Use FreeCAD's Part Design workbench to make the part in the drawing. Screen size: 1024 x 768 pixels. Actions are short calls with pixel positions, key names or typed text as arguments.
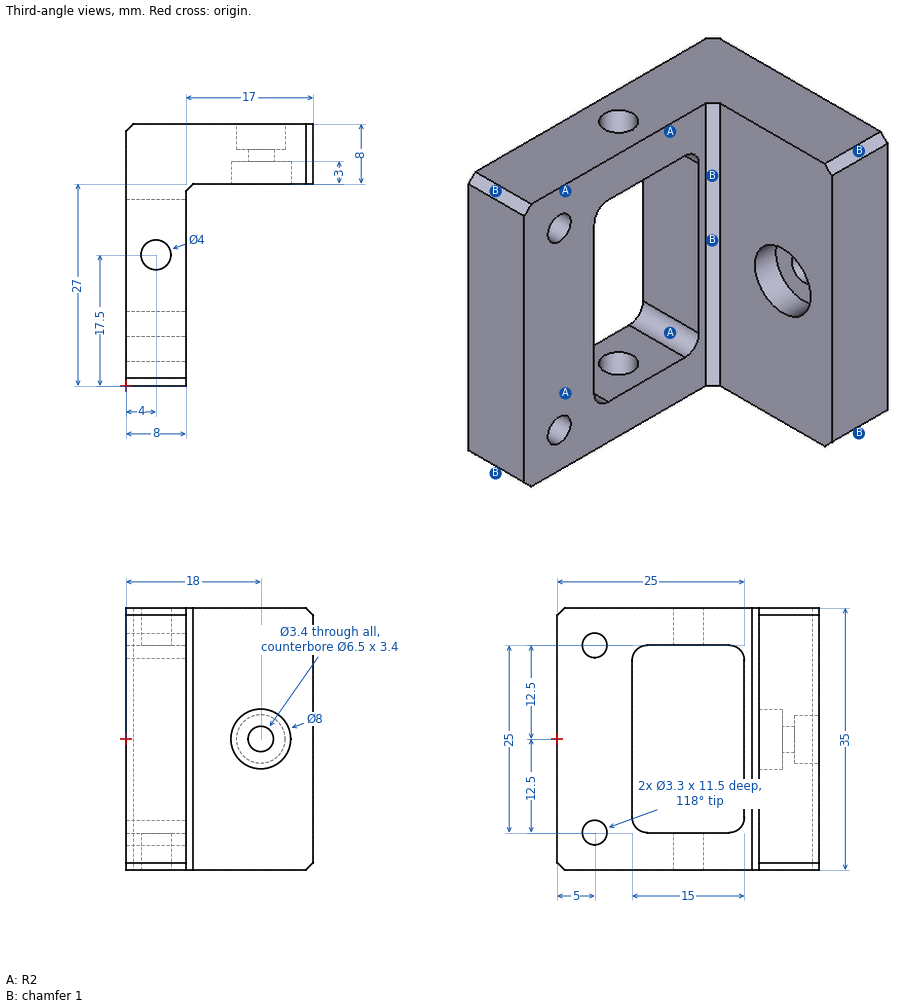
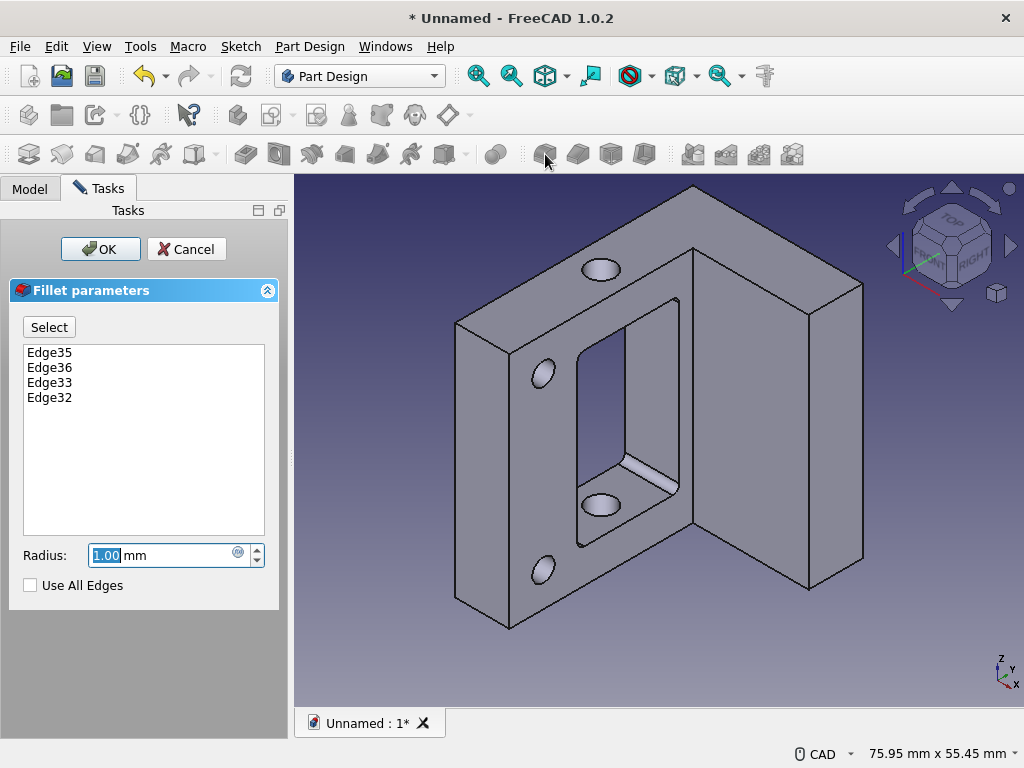
text(2)
key(Tab)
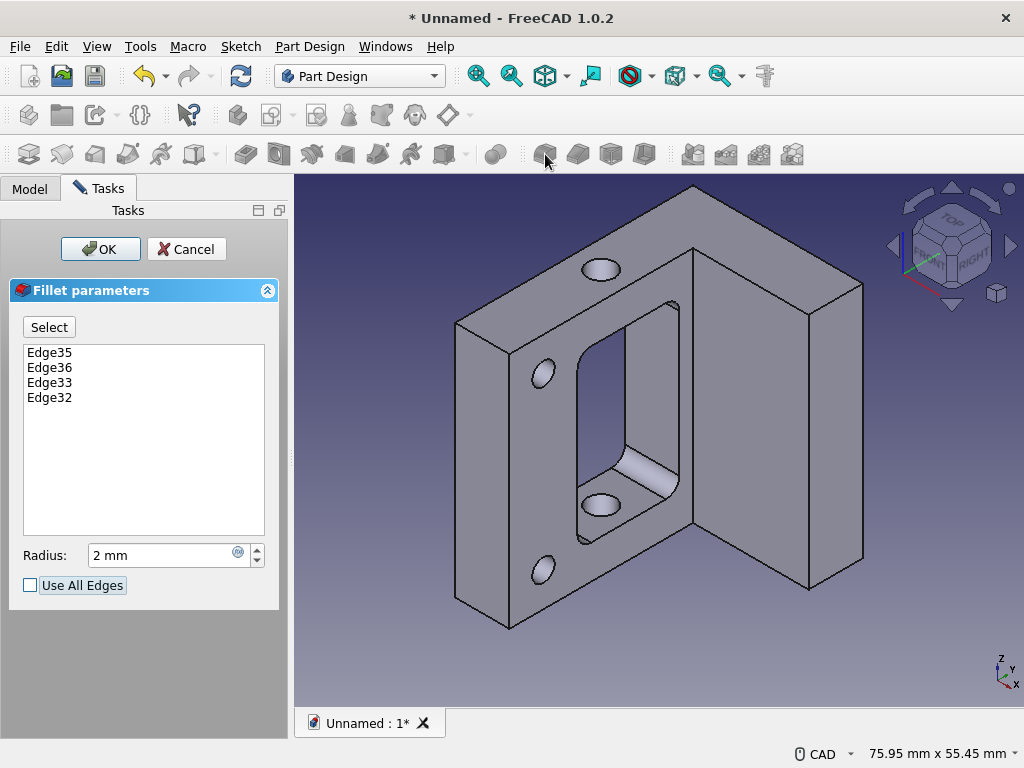
click(101, 249)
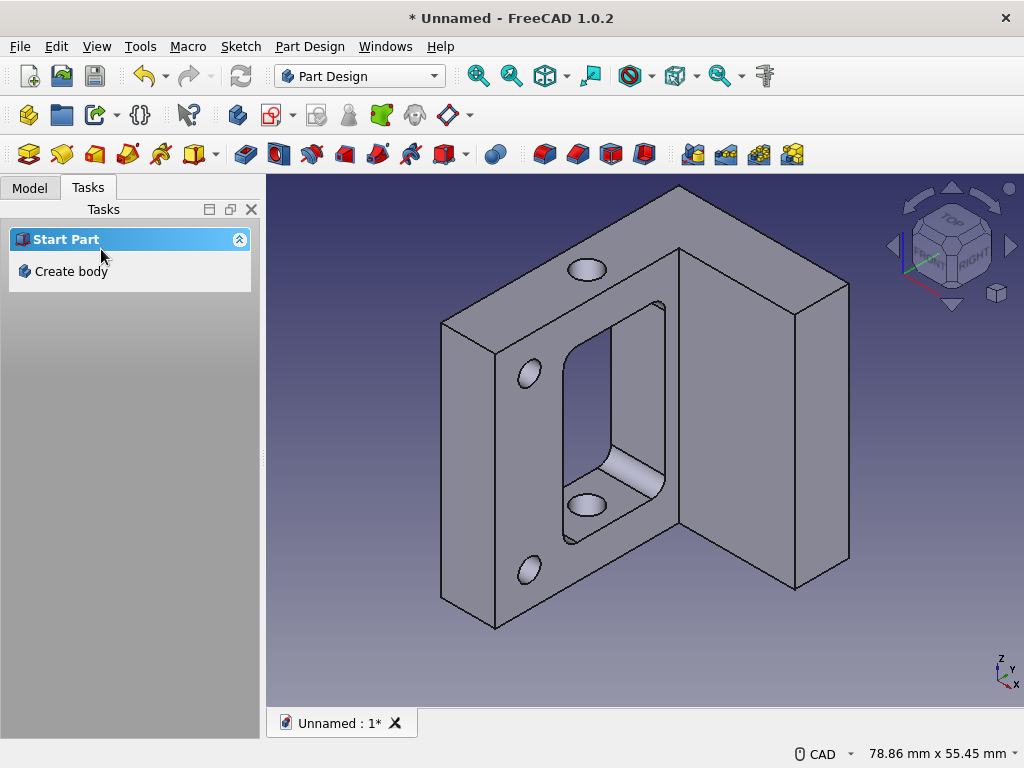
click(737, 379)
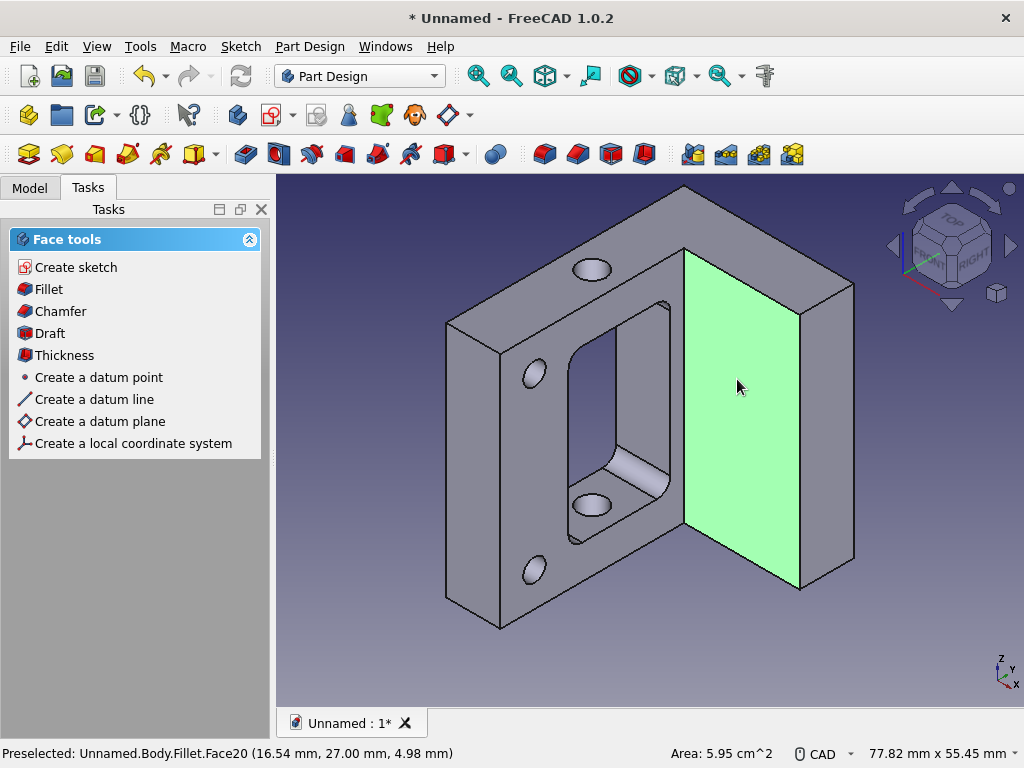
click(270, 116)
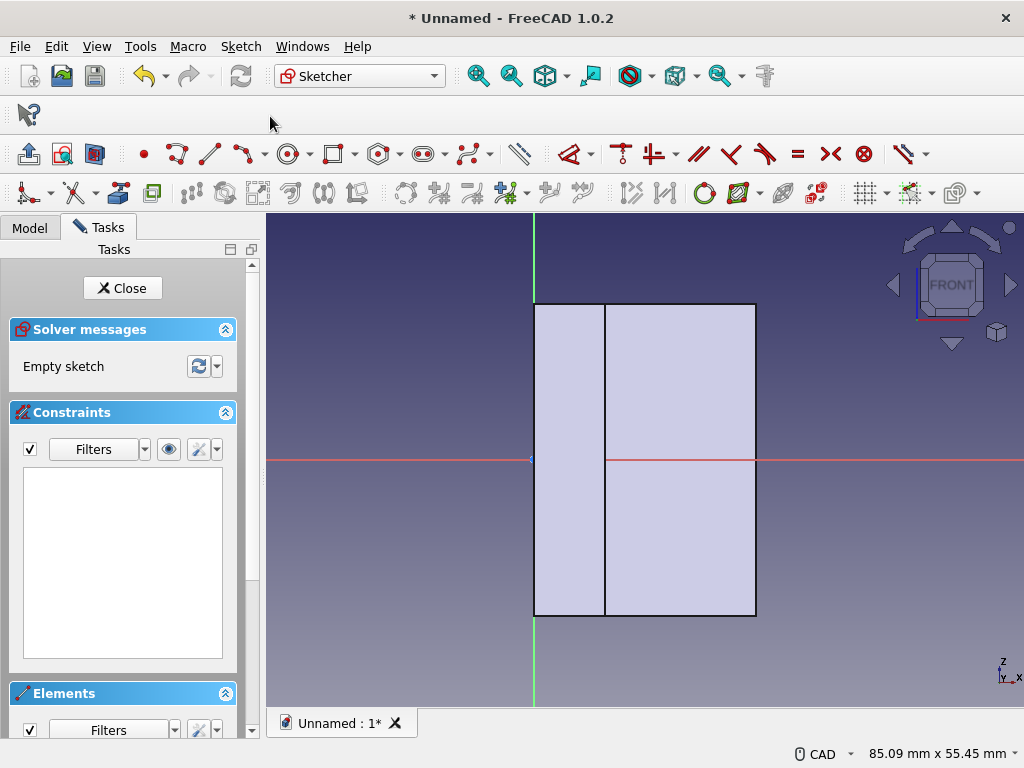
scroll(732, 460, up, 7)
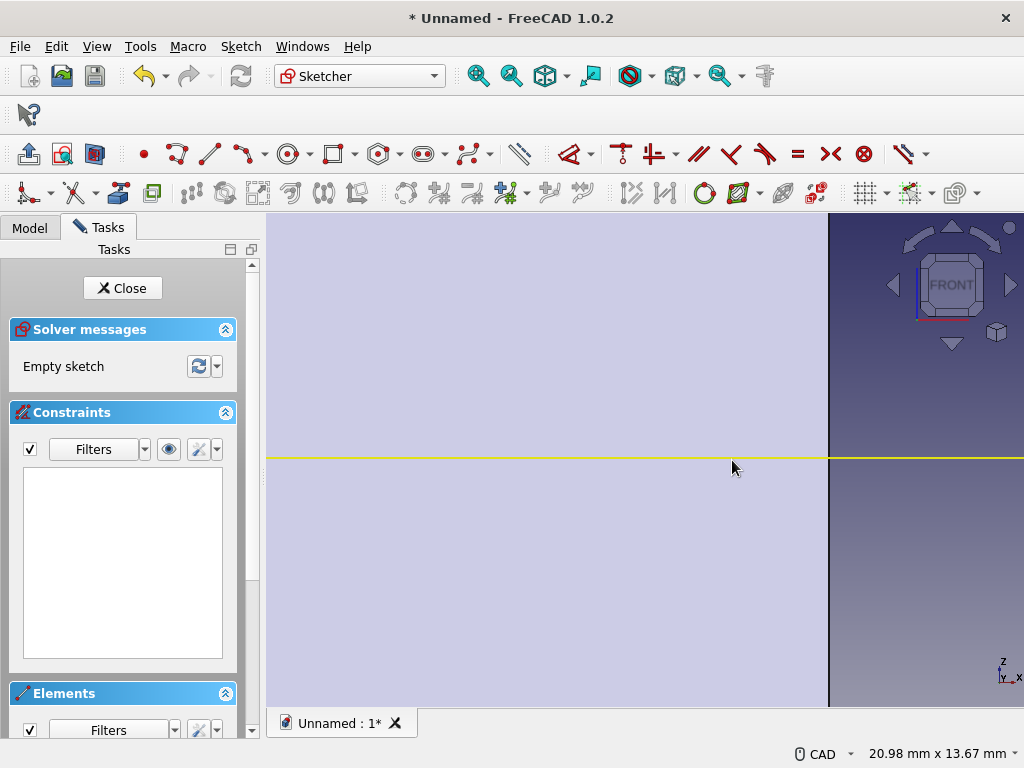
key(g)
key(c)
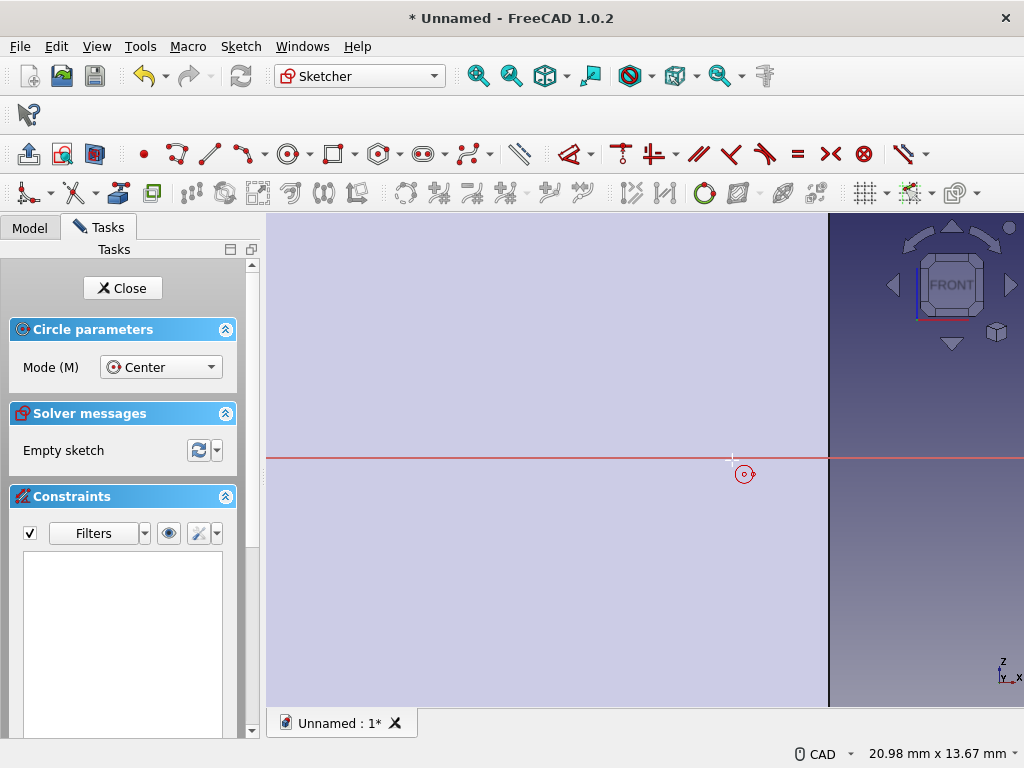
click(576, 458)
move(678, 356)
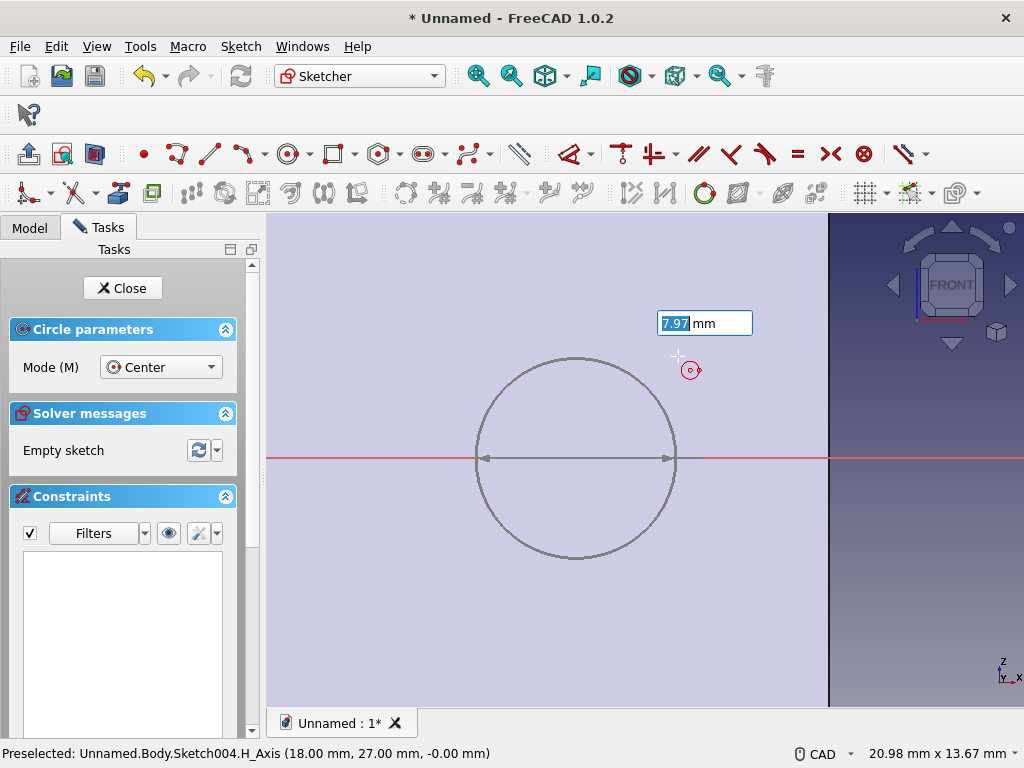
text(8)
key(Return)
key(Escape)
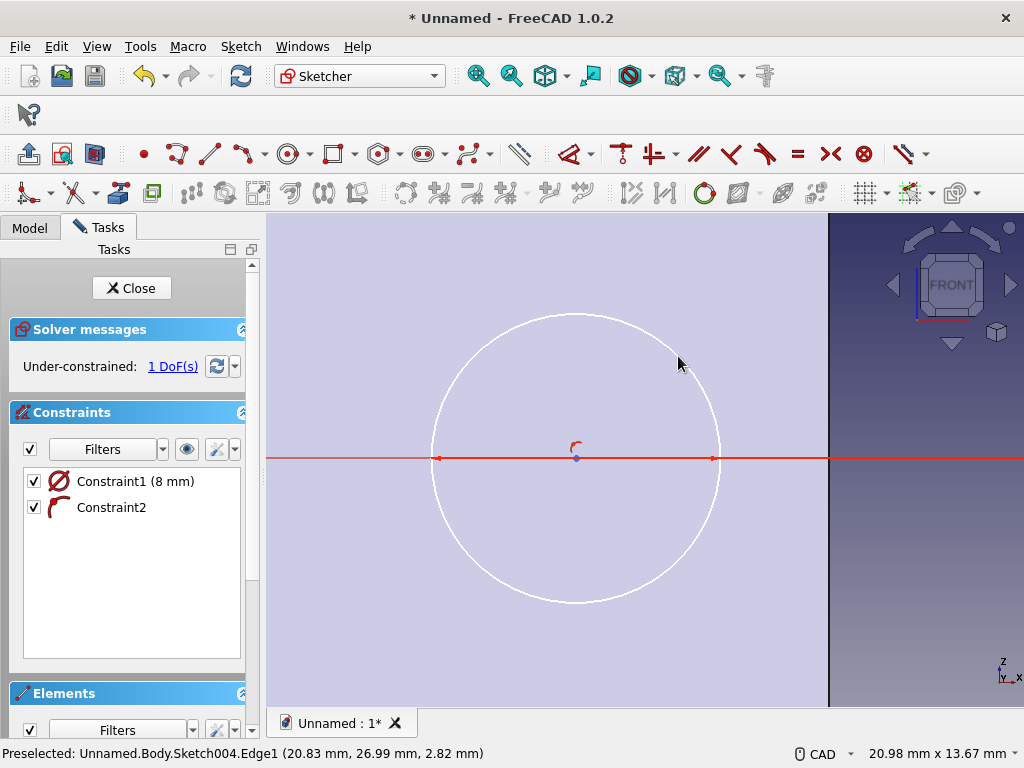
key(d)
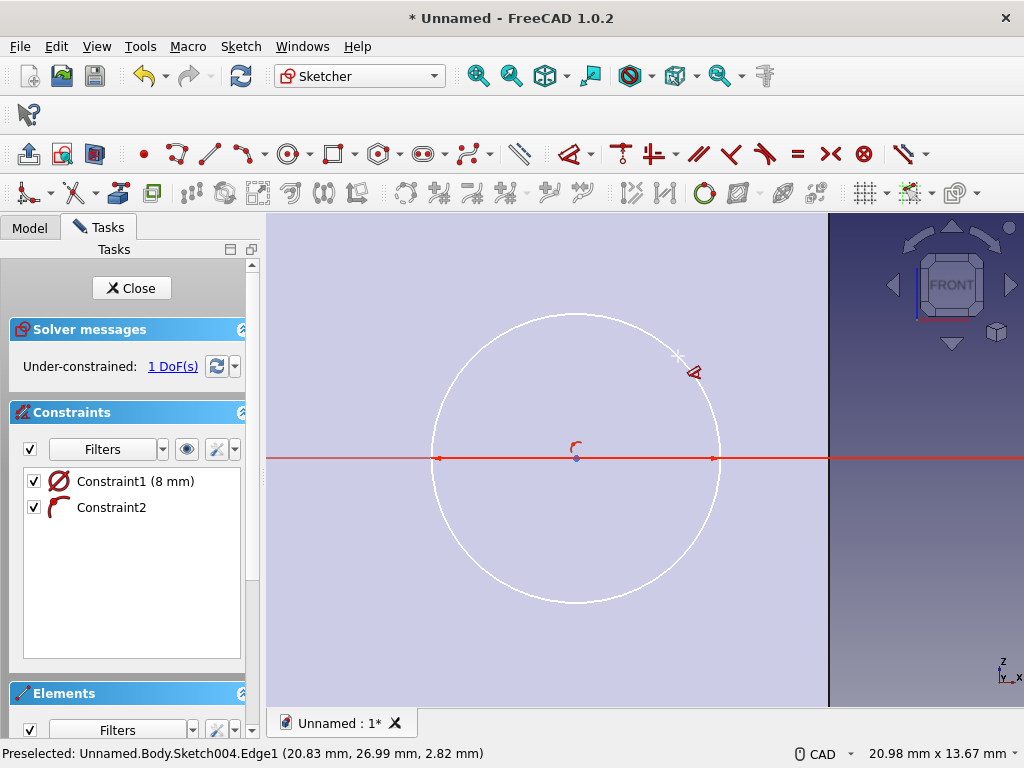
click(576, 458)
click(370, 492)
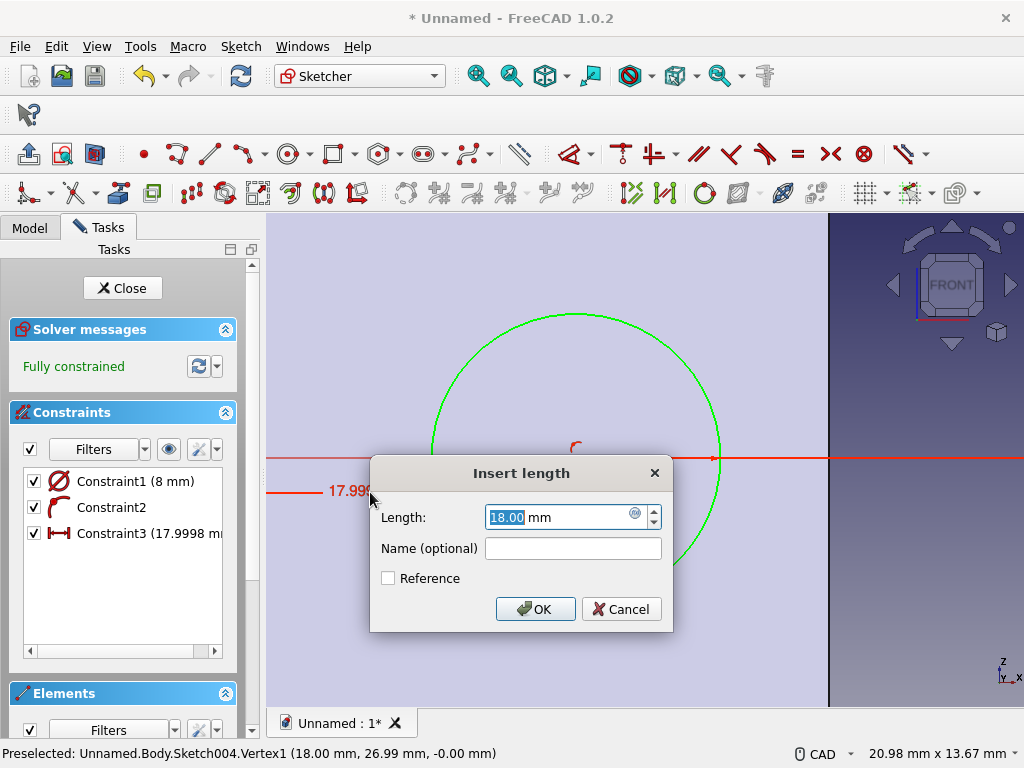
text(18)
key(Return)
key(Escape)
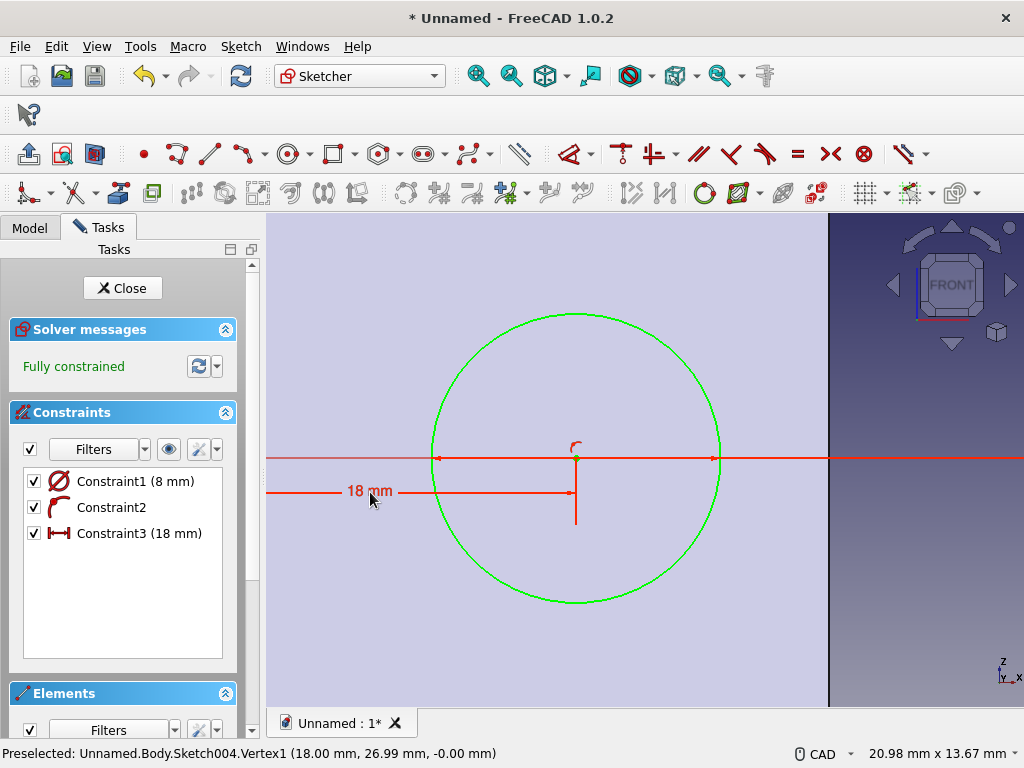
click(123, 288)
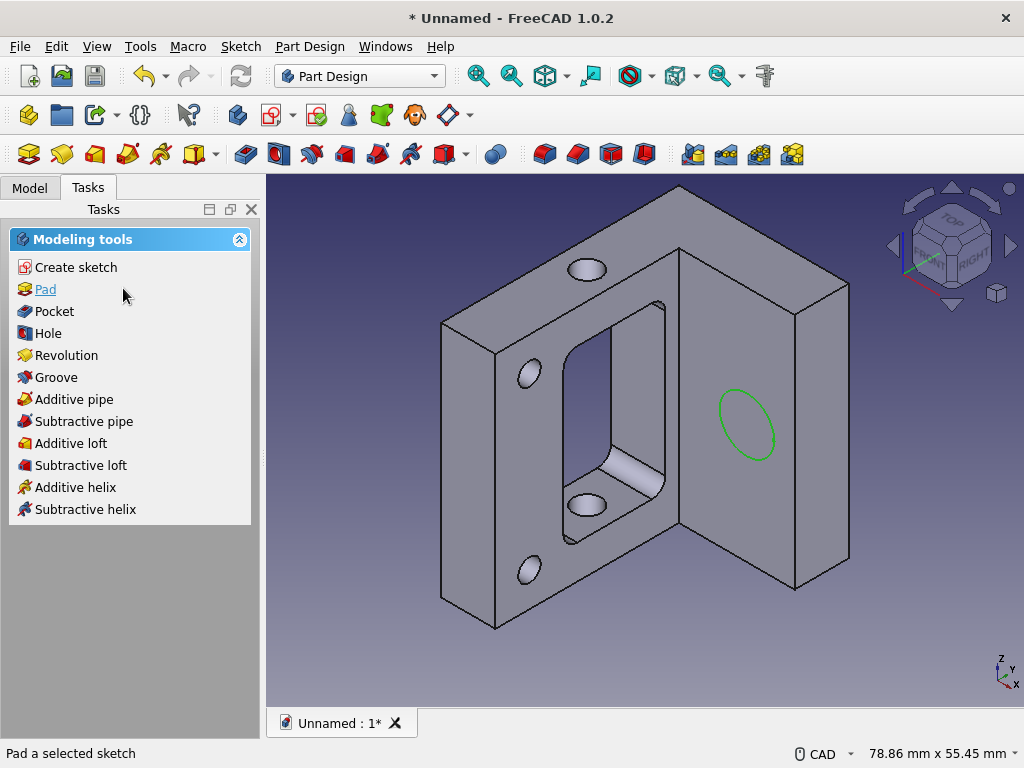
click(246, 154)